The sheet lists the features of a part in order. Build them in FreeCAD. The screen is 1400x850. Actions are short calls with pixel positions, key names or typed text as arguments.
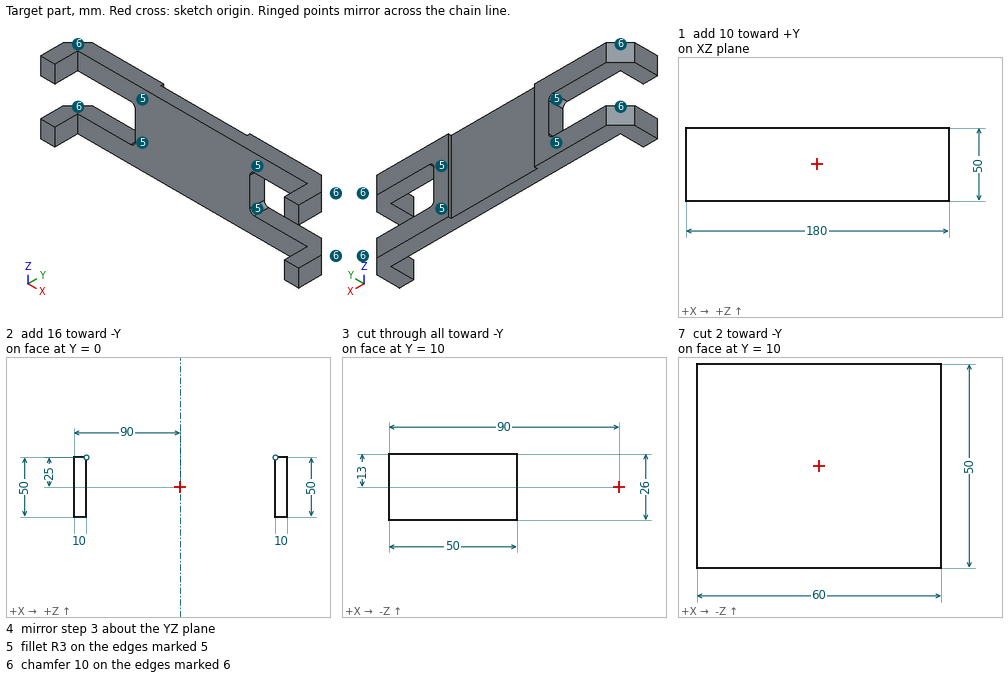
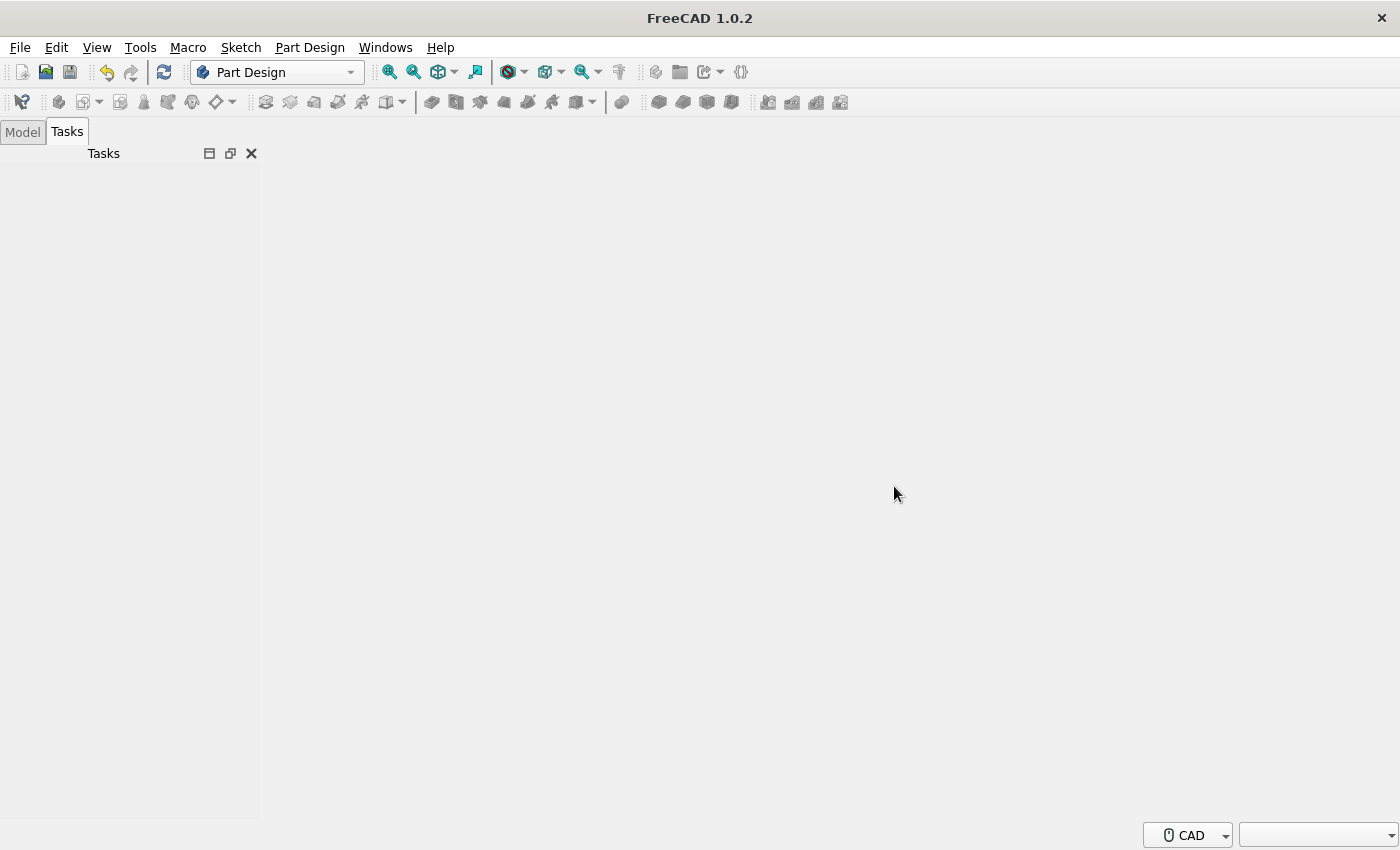
click(22, 72)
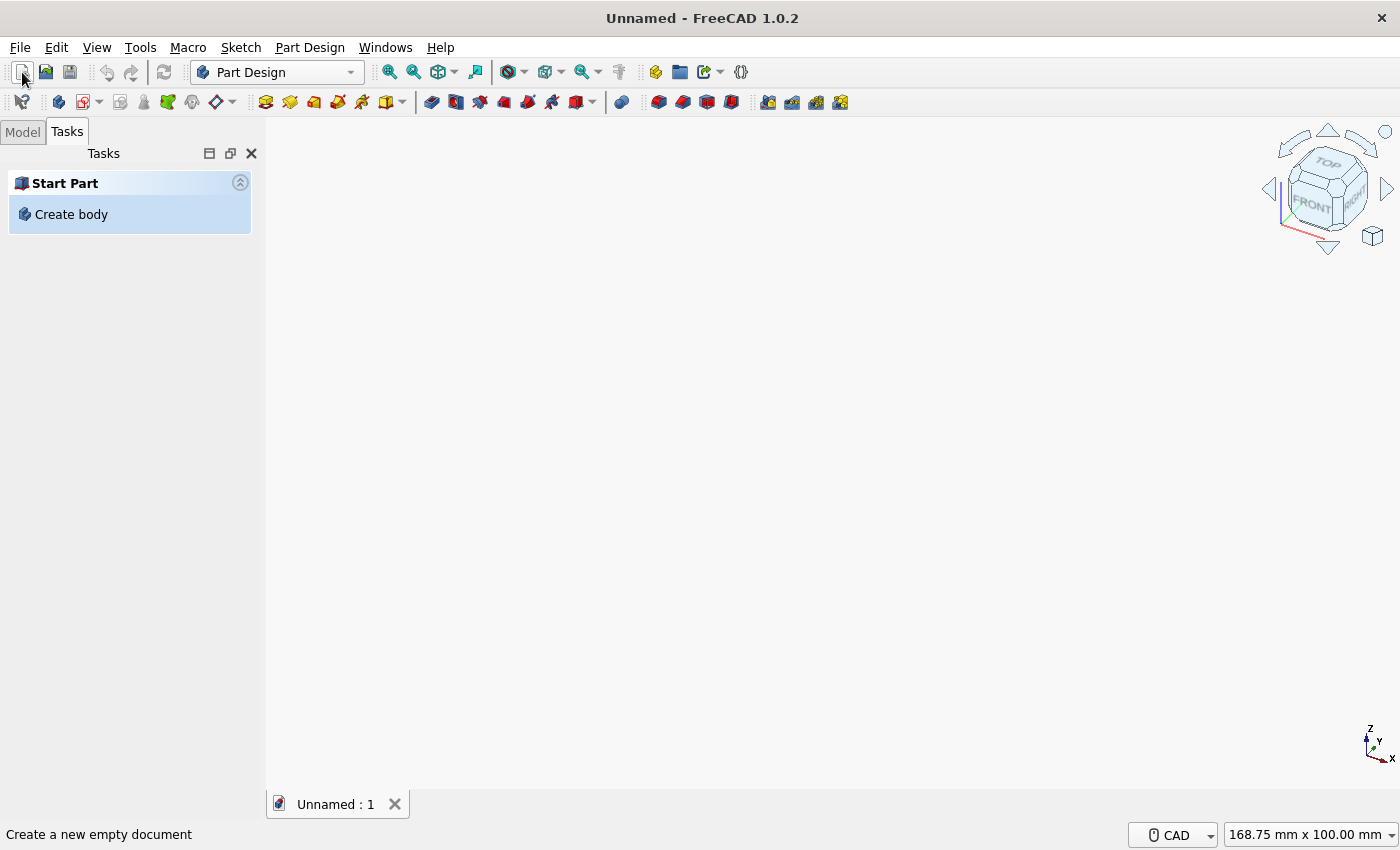
click(84, 102)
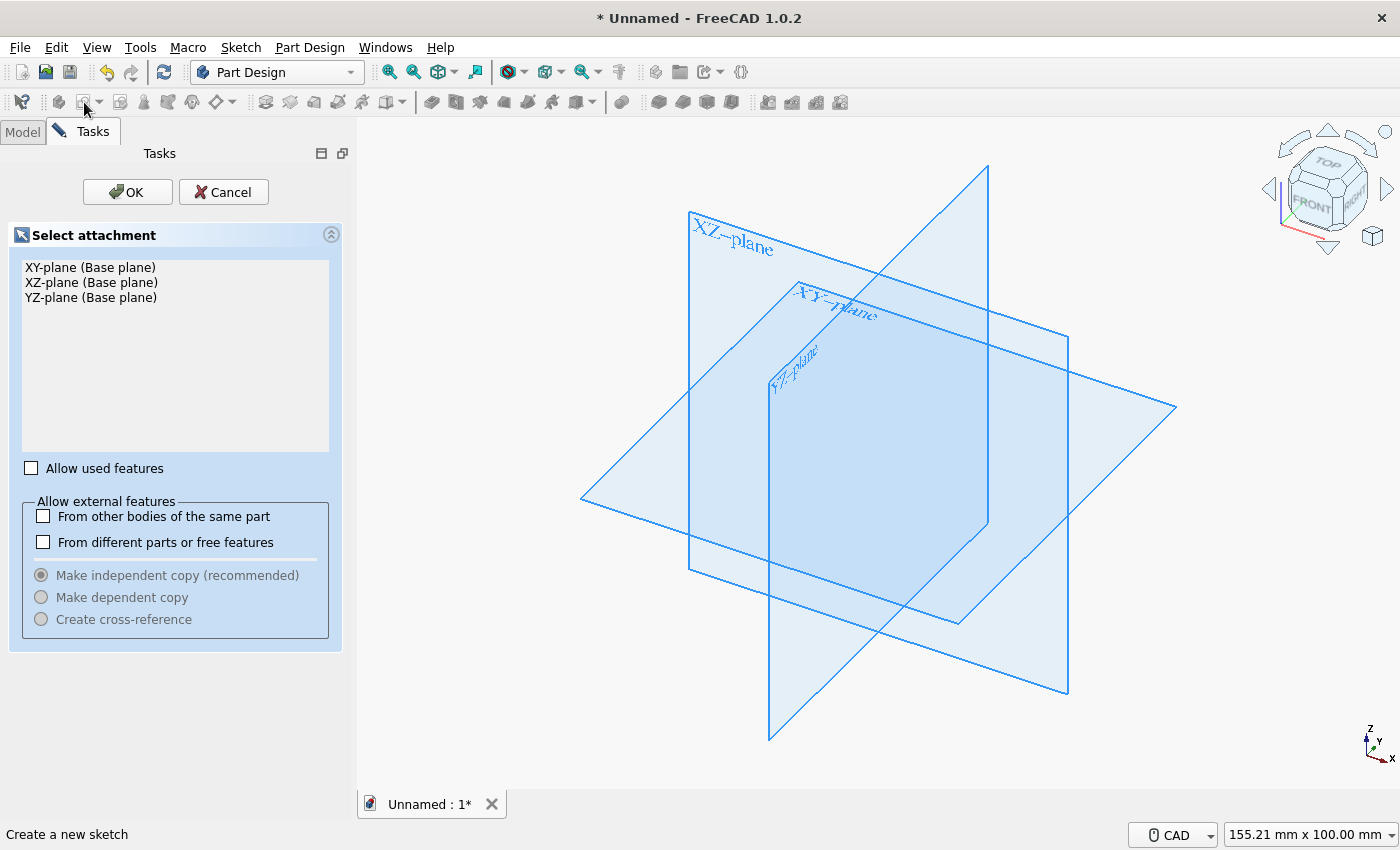
click(82, 282)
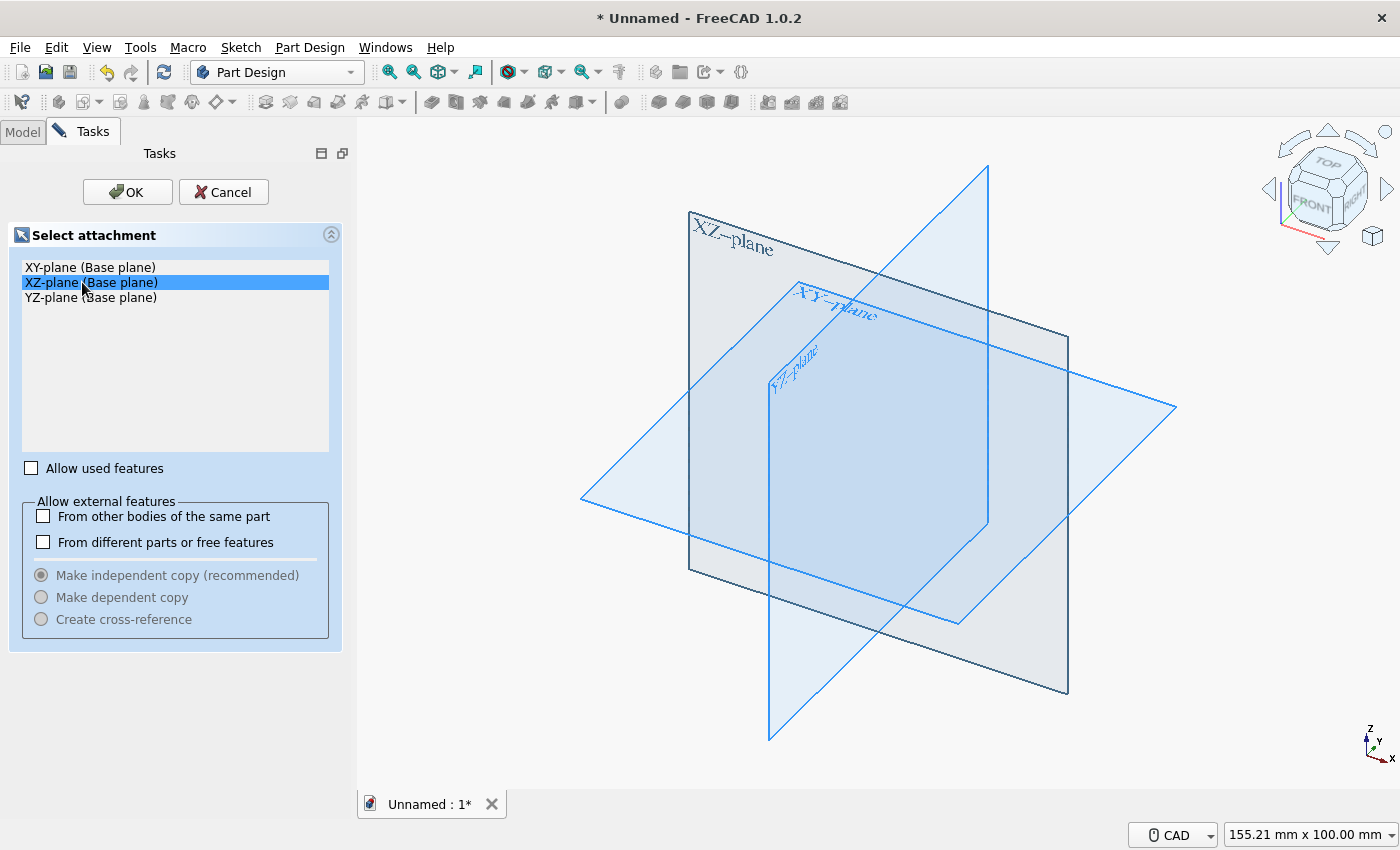
click(128, 192)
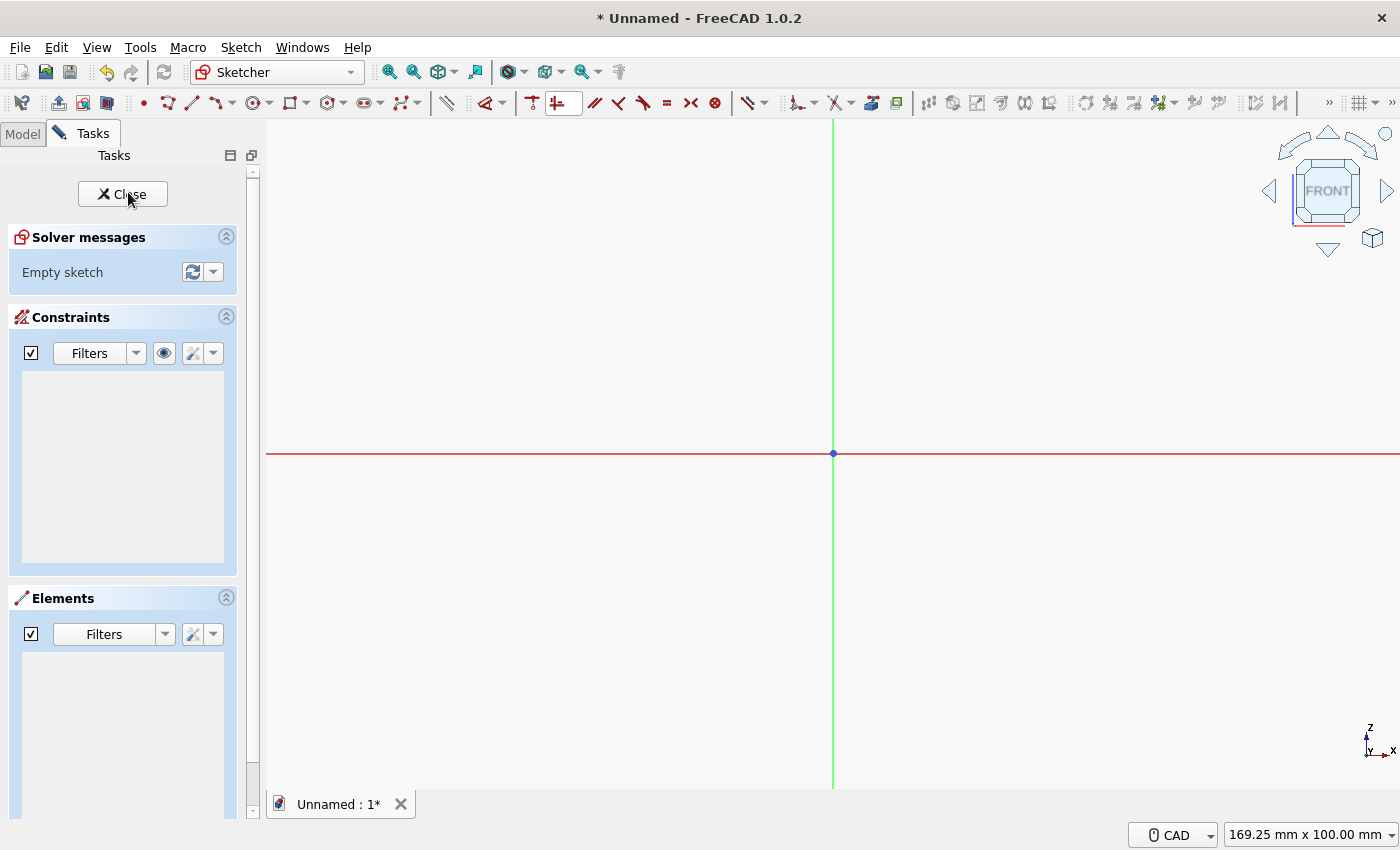
scroll(681, 454, down, 3)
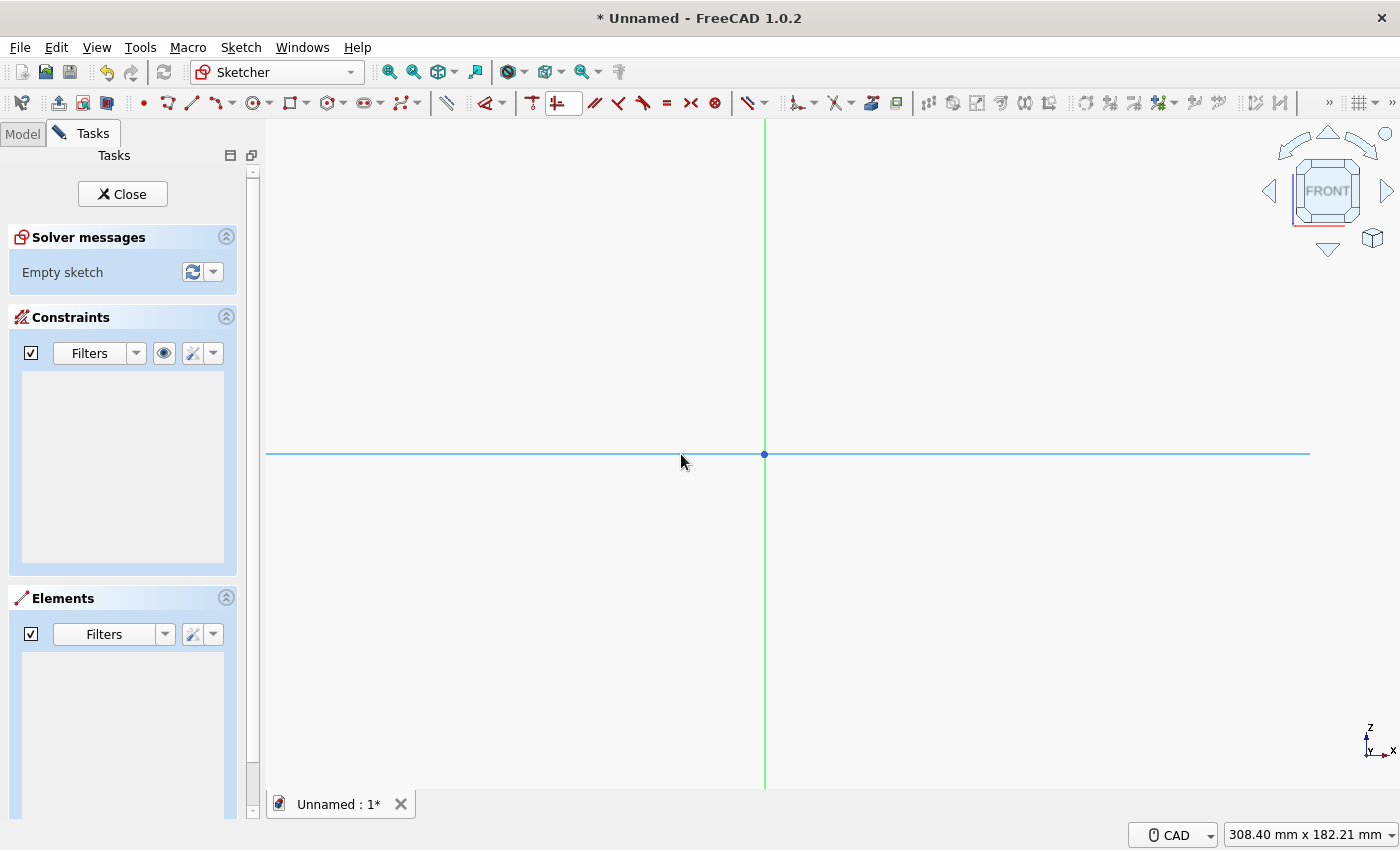
key(g)
key(v)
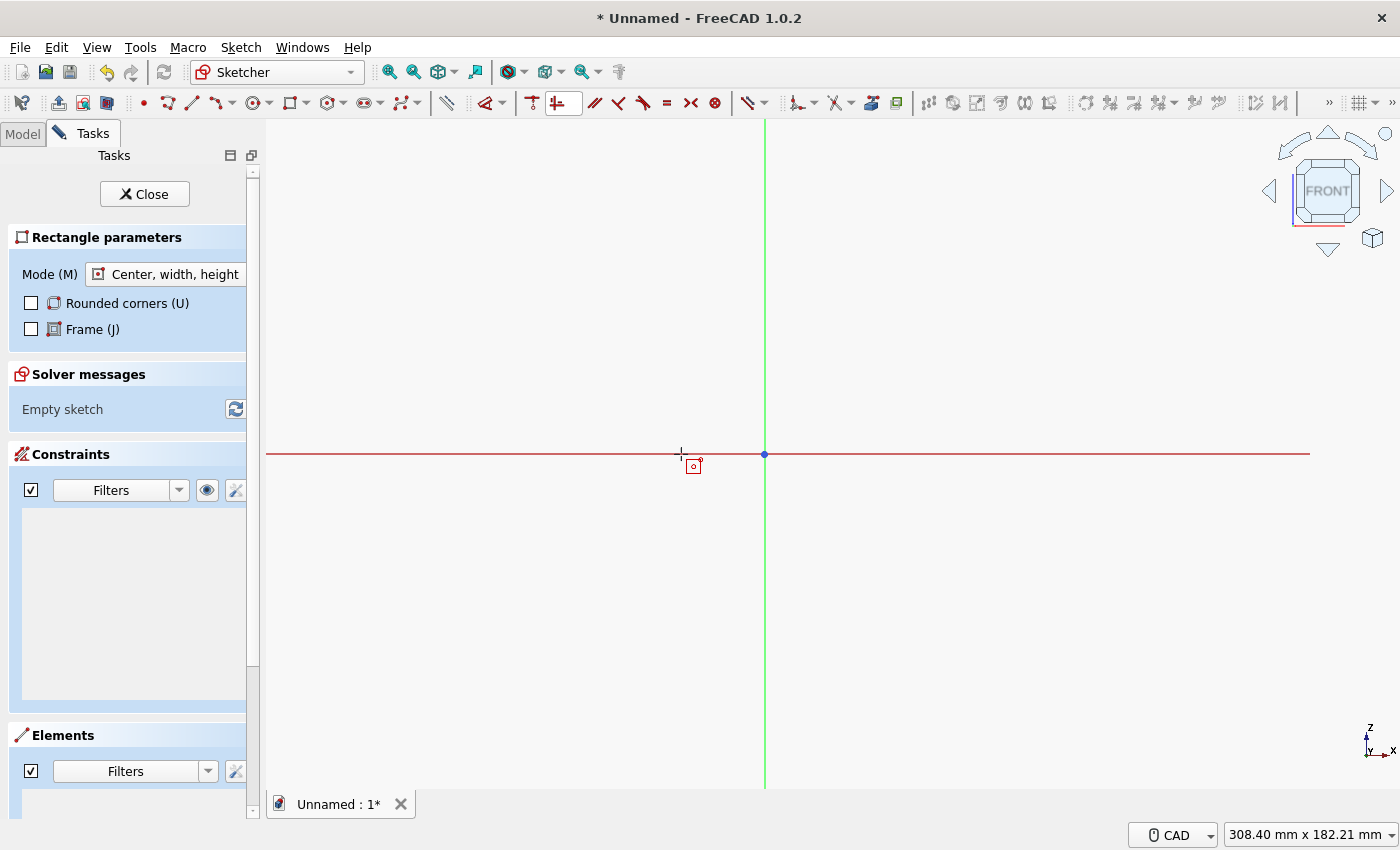
click(765, 454)
move(1096, 362)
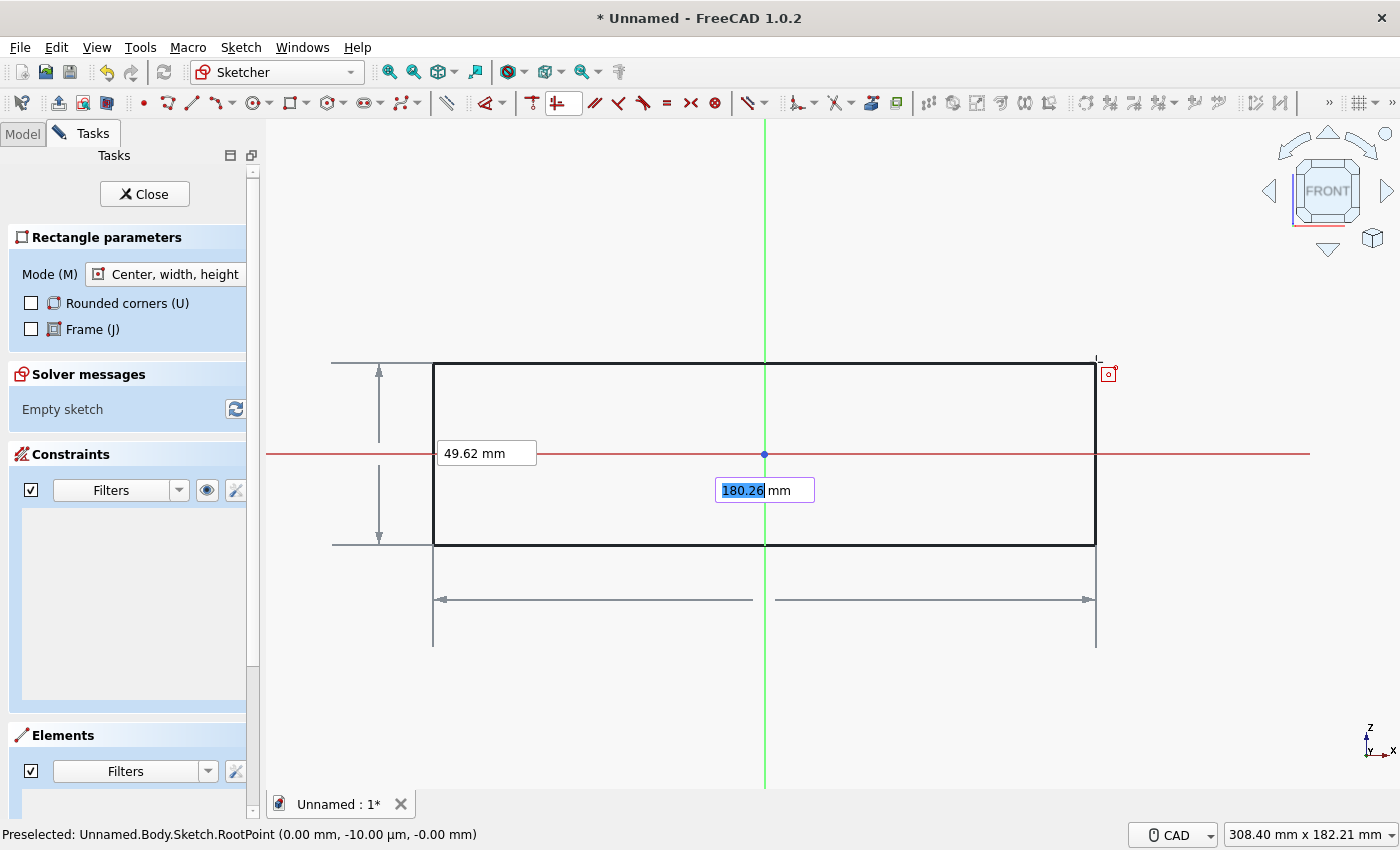
text(180)
key(Tab)
text(50)
key(Return)
key(Escape)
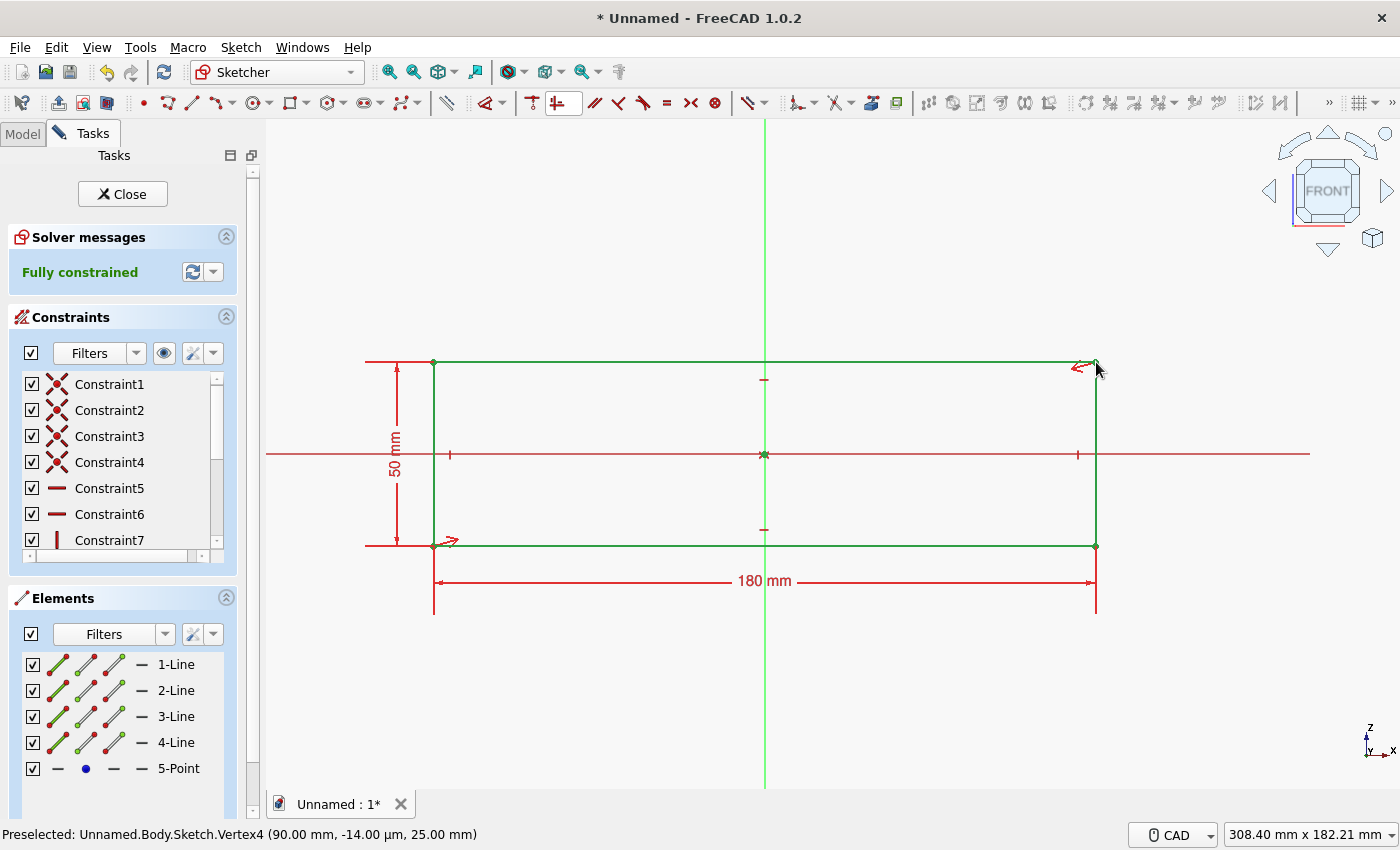
click(123, 194)